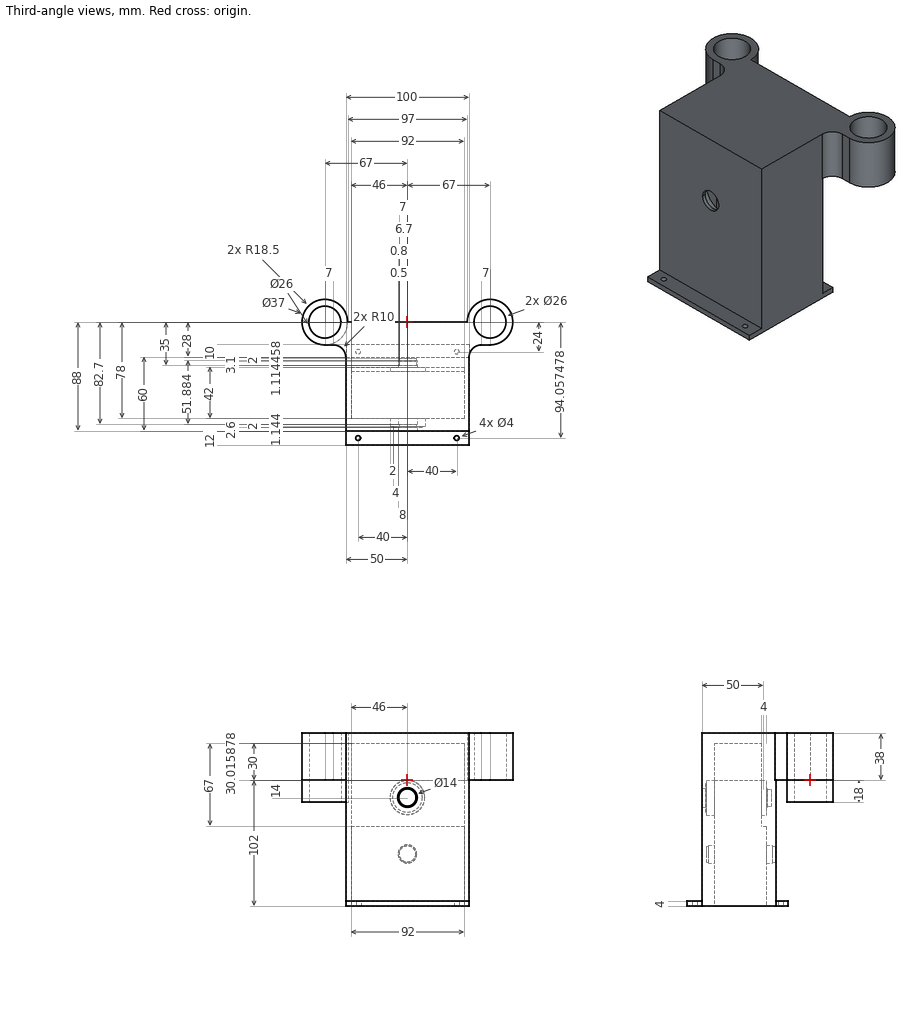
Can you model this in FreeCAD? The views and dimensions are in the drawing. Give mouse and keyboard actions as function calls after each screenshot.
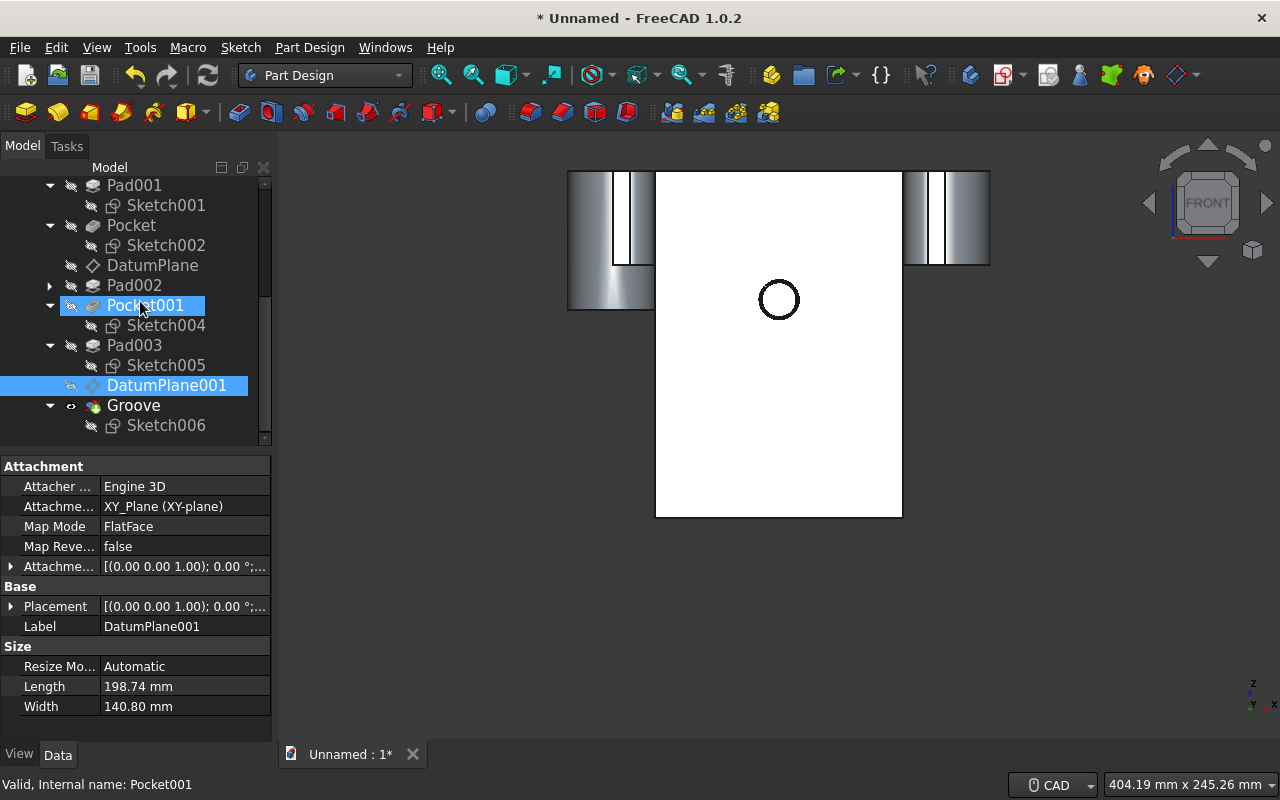
scroll(140, 301, up, 15)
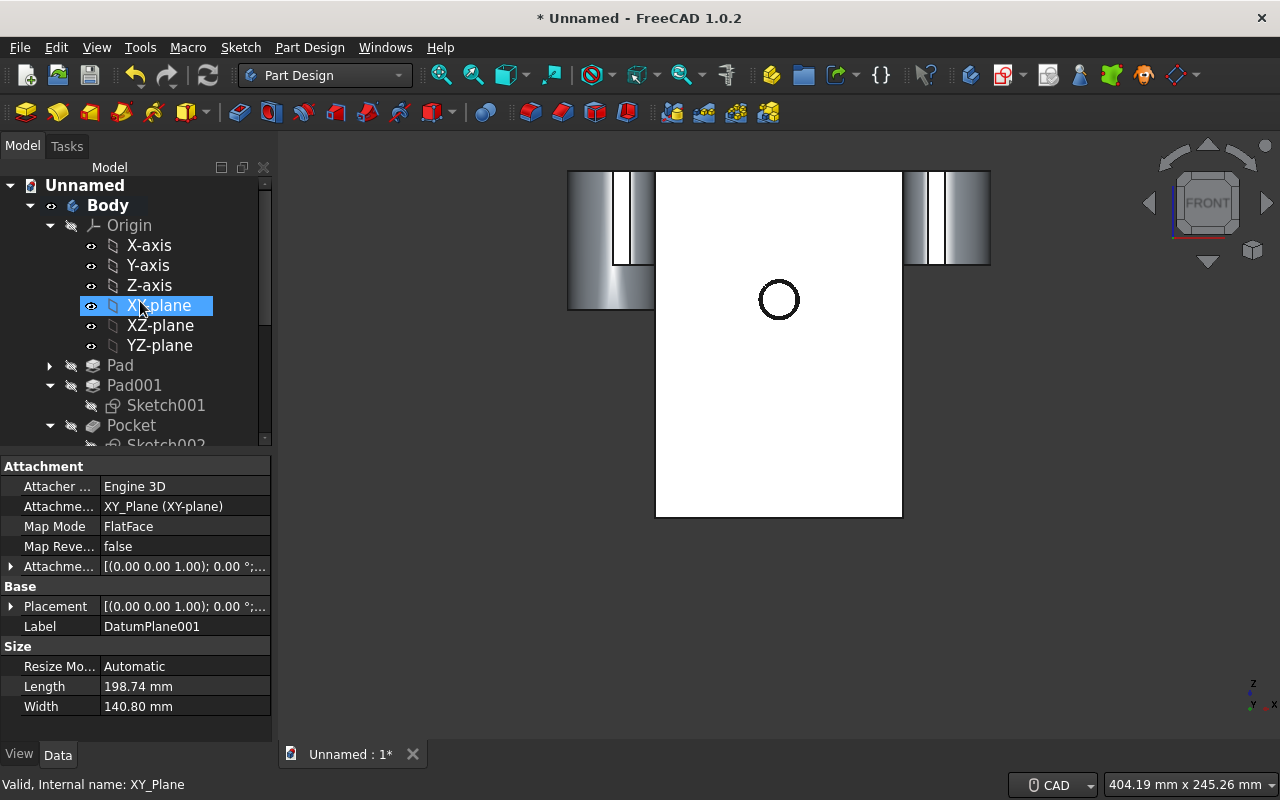
click(136, 306)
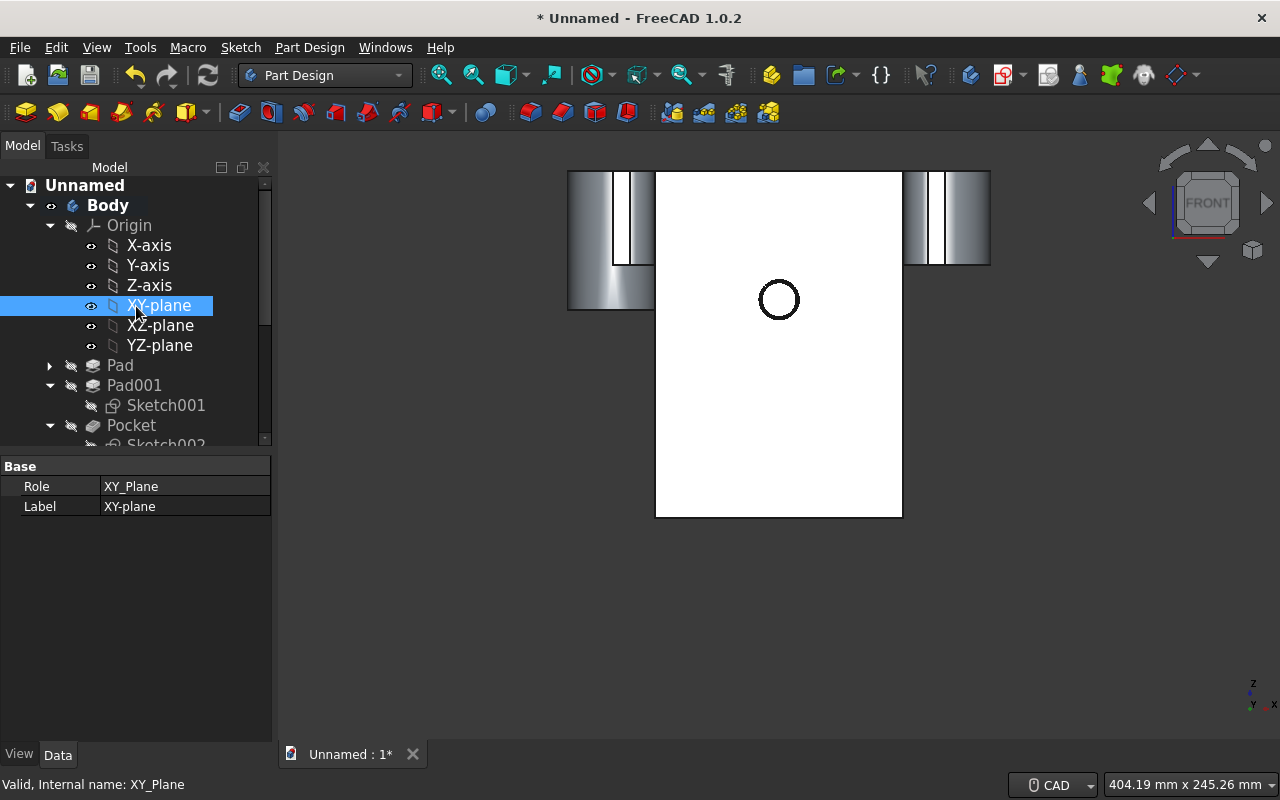
click(1176, 76)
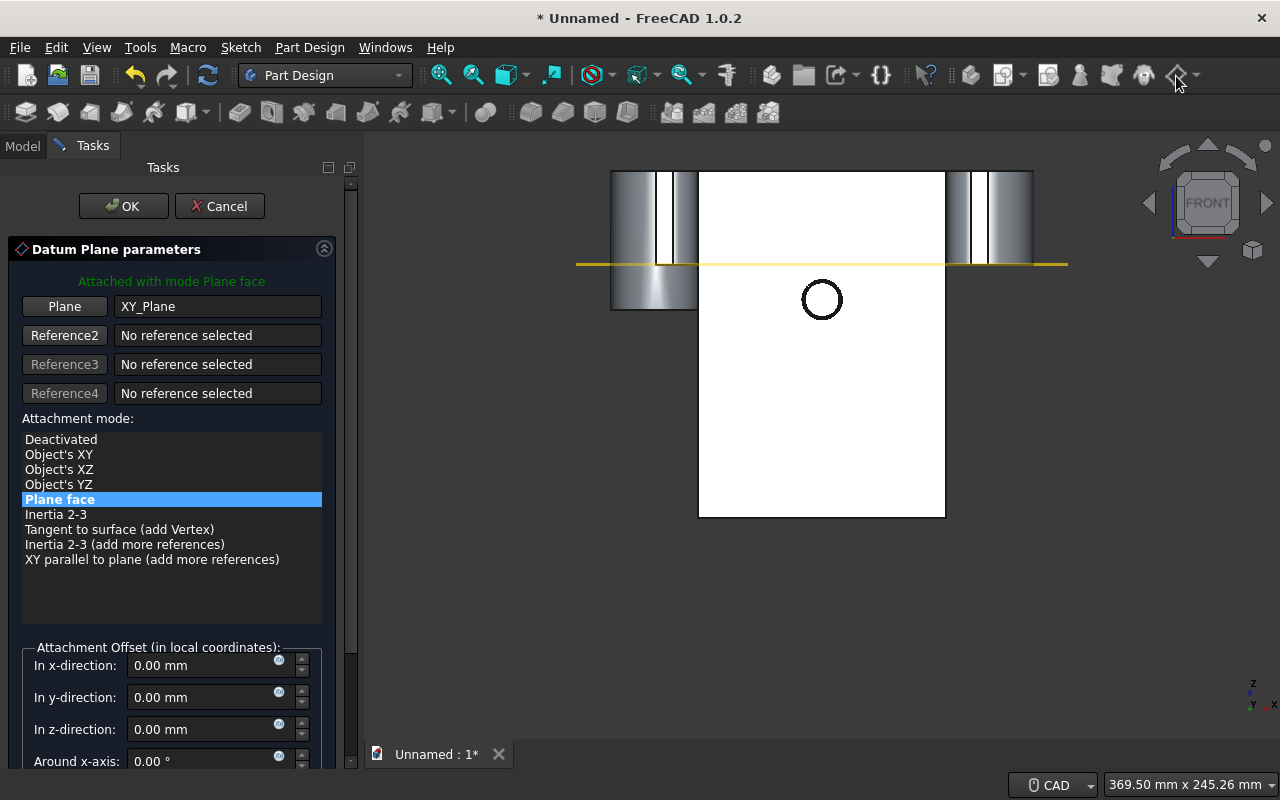
triple_click(210, 729)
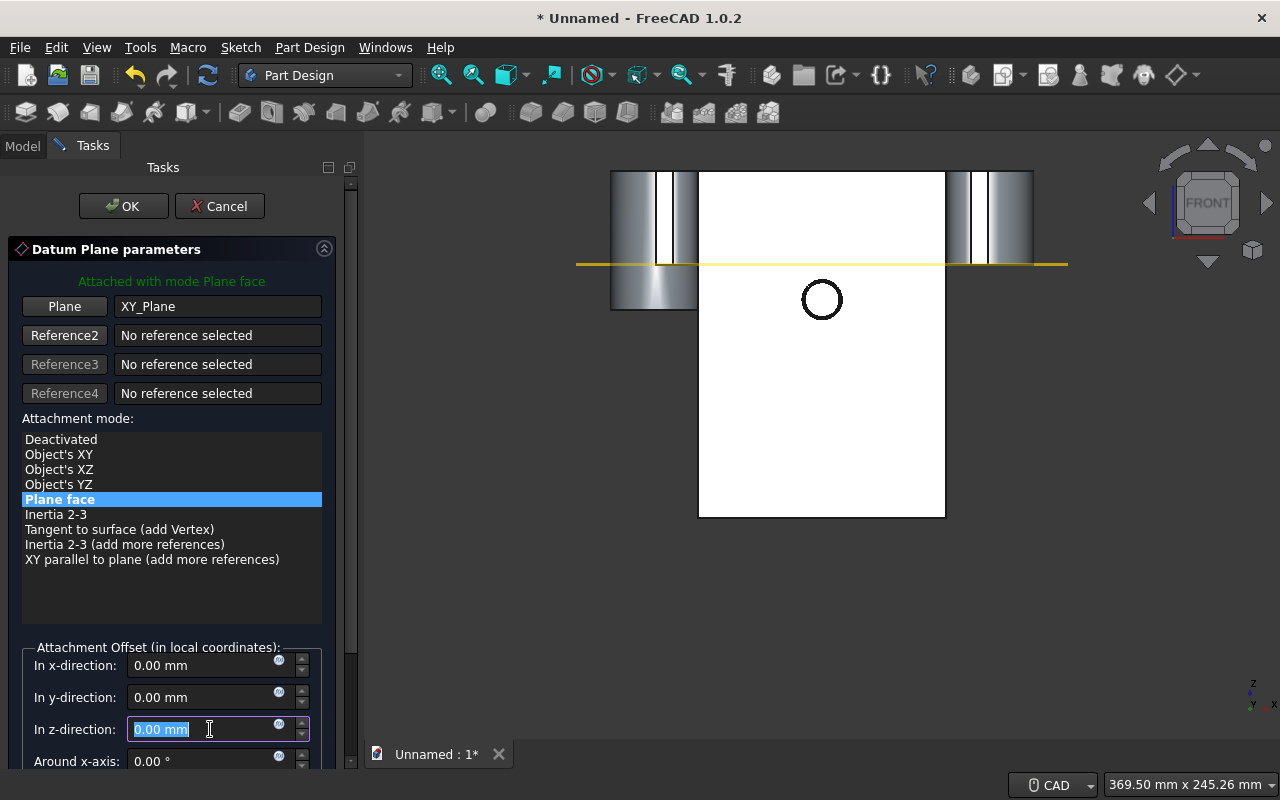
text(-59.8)
key(Tab)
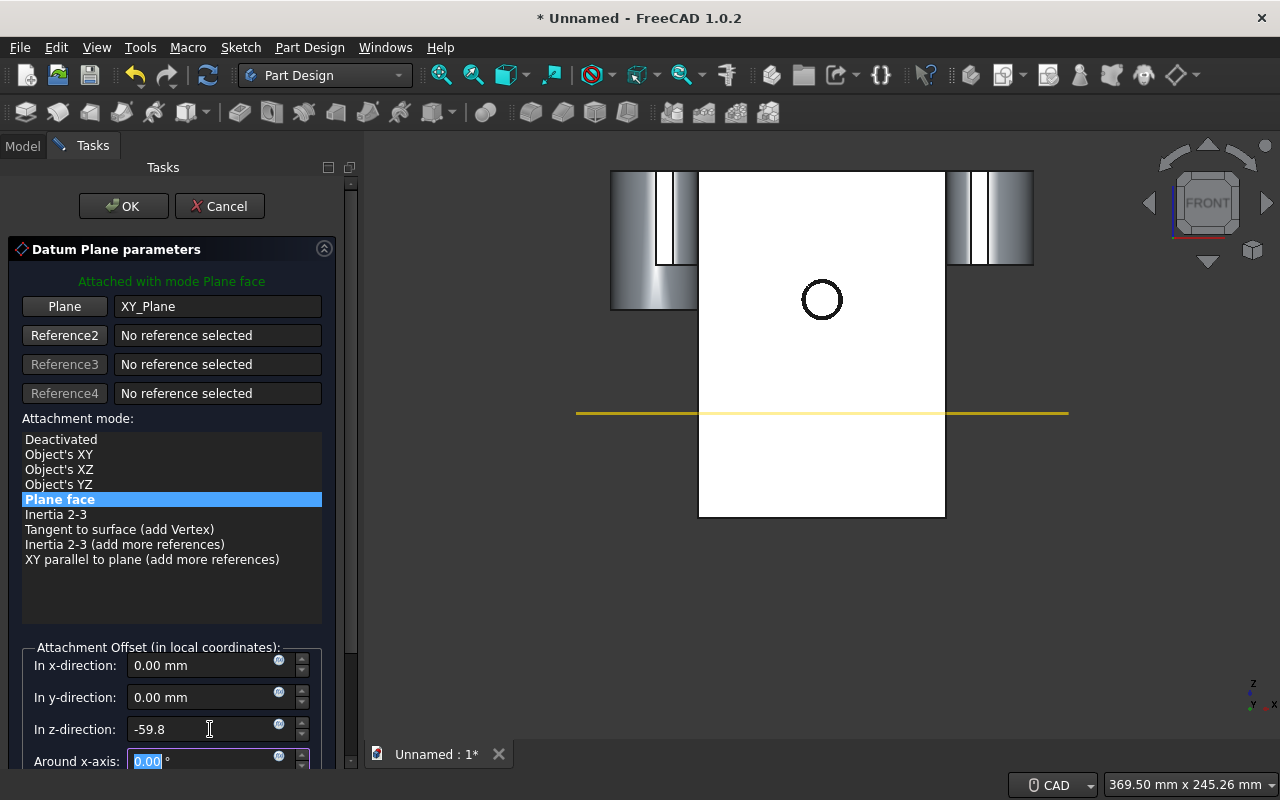
click(124, 206)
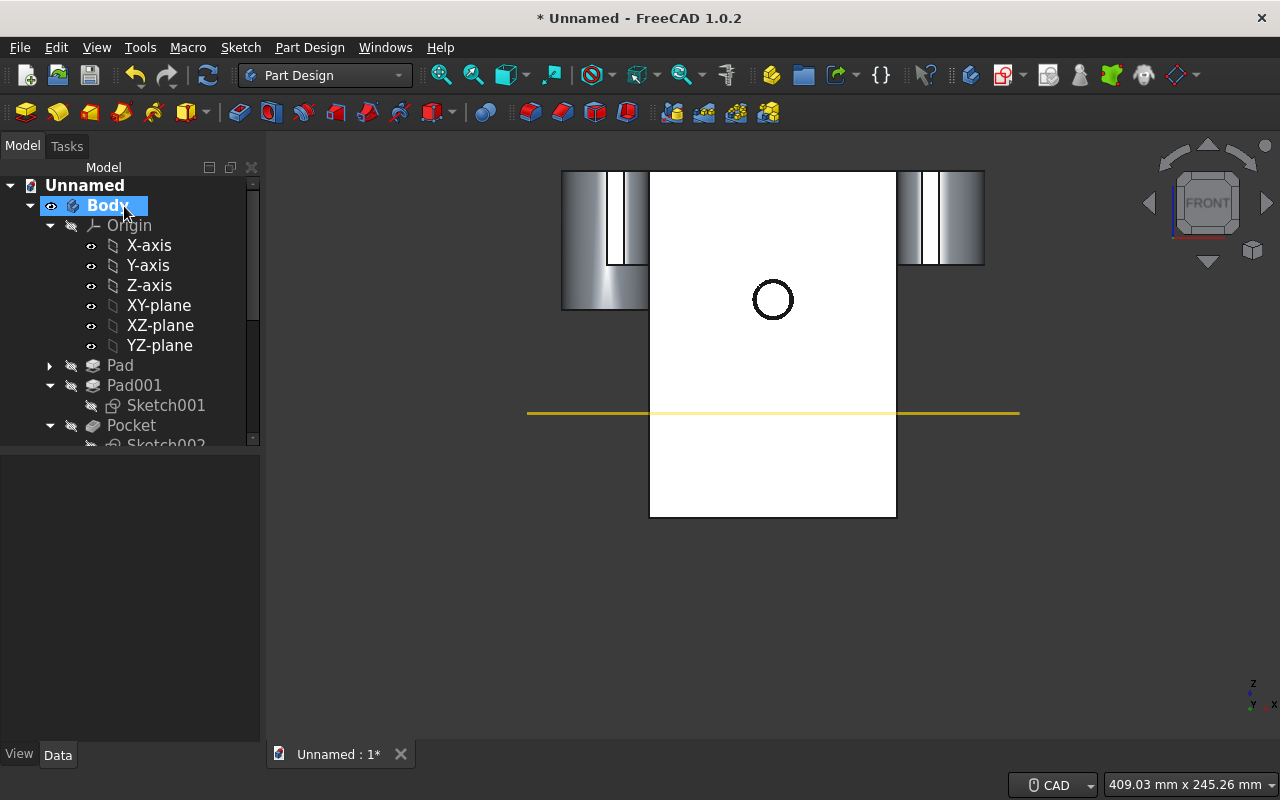
scroll(100, 321, down, 3)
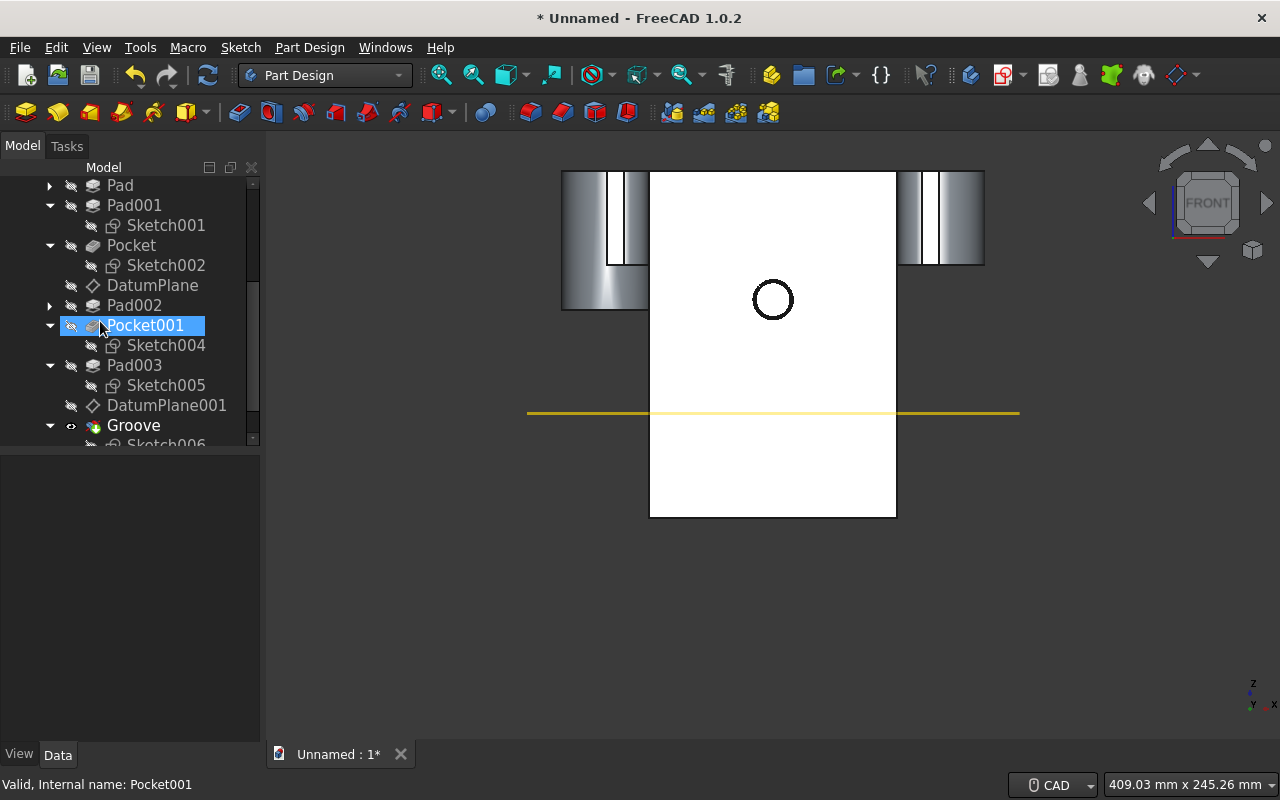
scroll(140, 321, up, 15)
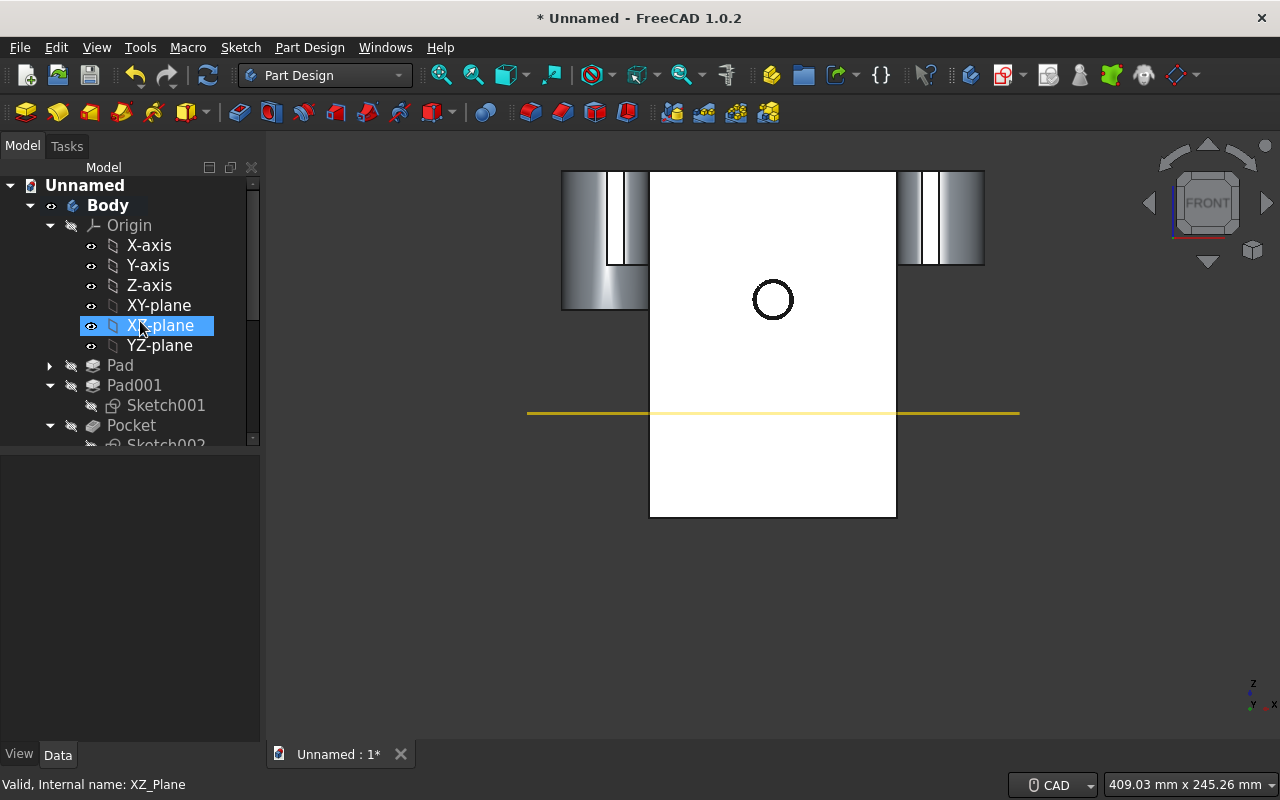
scroll(100, 321, down, 6)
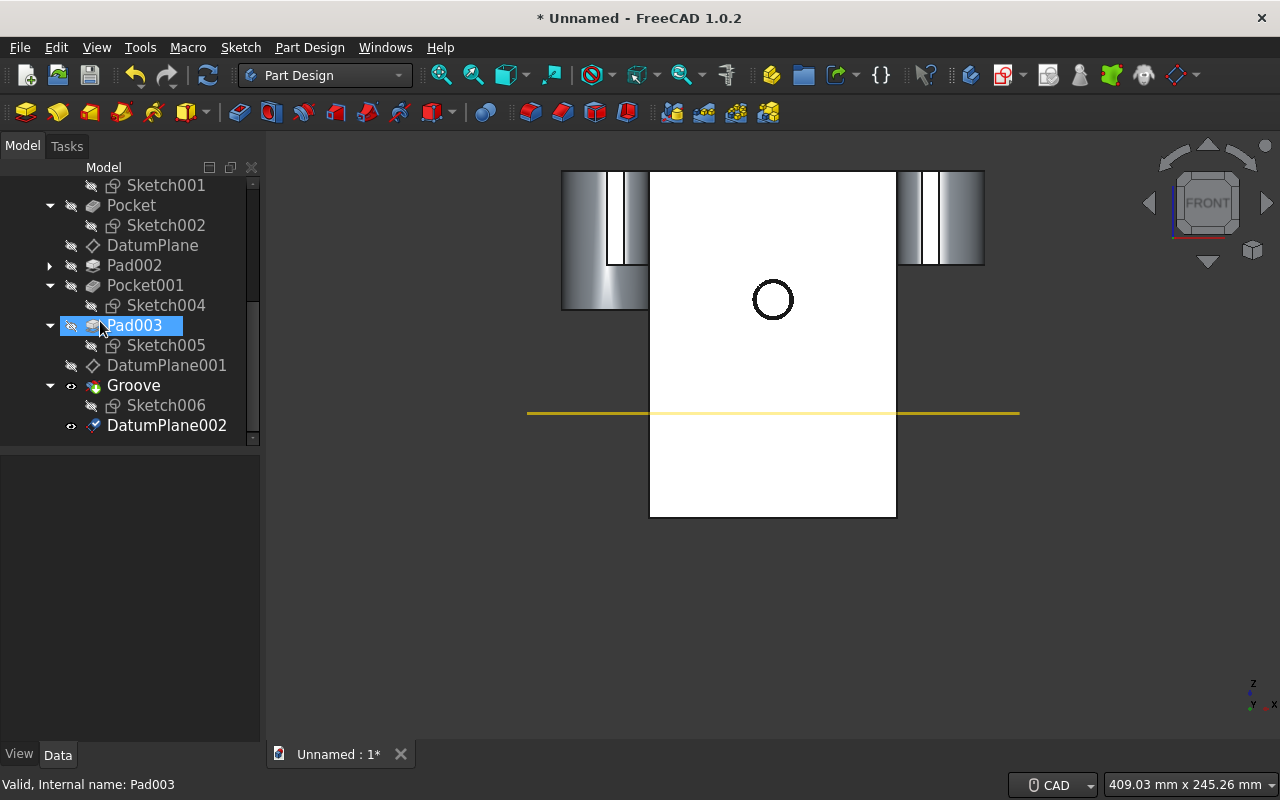
click(116, 426)